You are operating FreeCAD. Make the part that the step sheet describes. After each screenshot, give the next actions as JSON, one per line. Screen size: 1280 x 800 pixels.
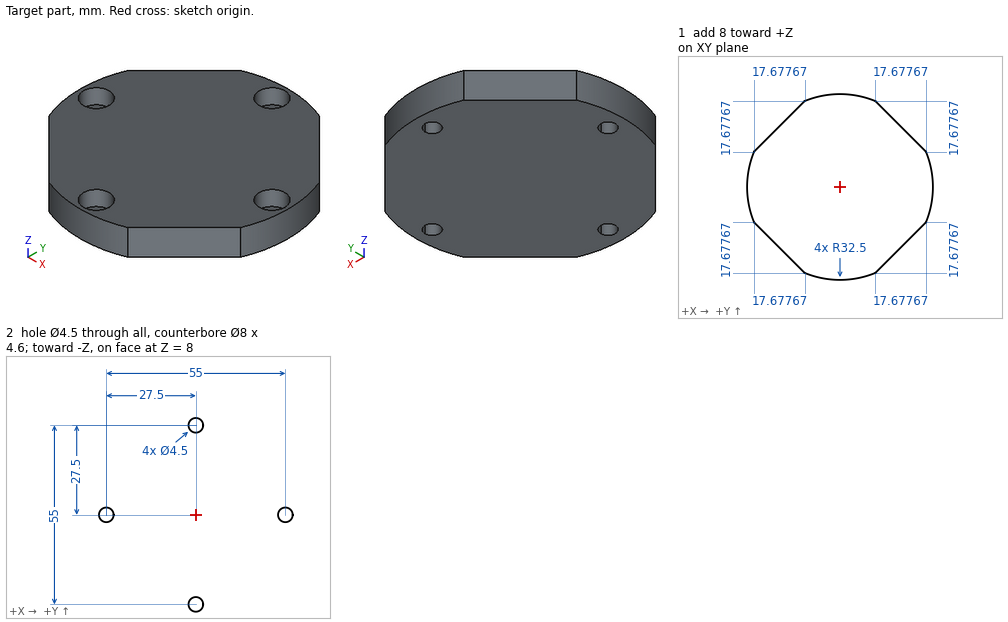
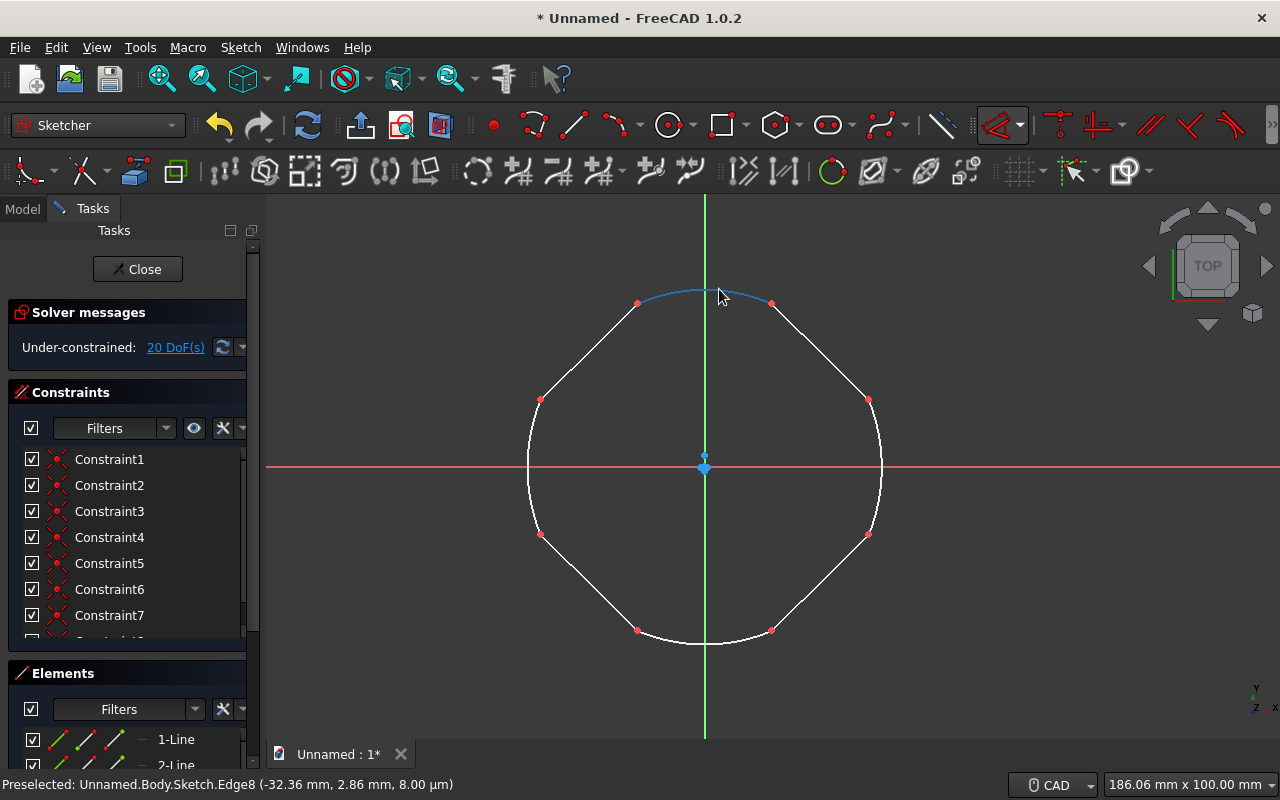
{"action": "left_click", "coordinate": [677, 642]}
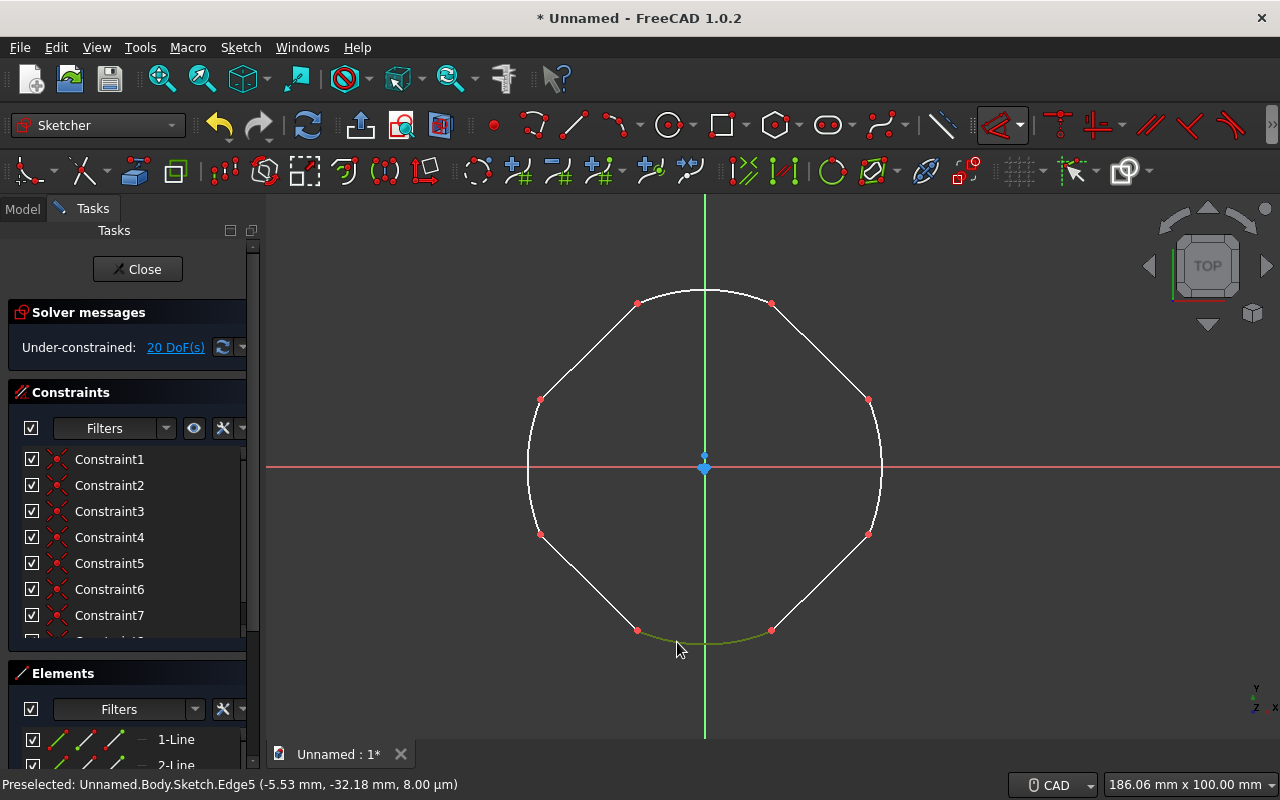
{"action": "left_click", "coordinate": [880, 495]}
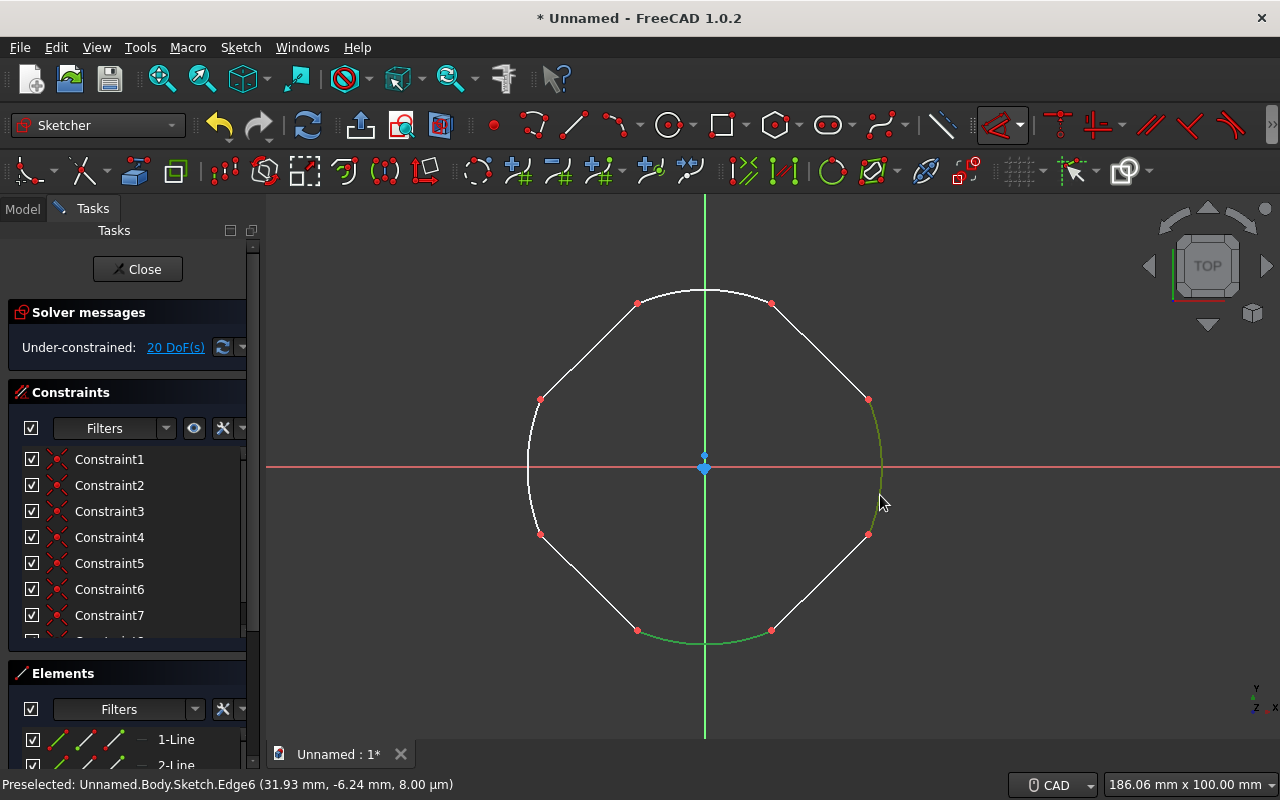
{"action": "left_click", "coordinate": [1058, 126]}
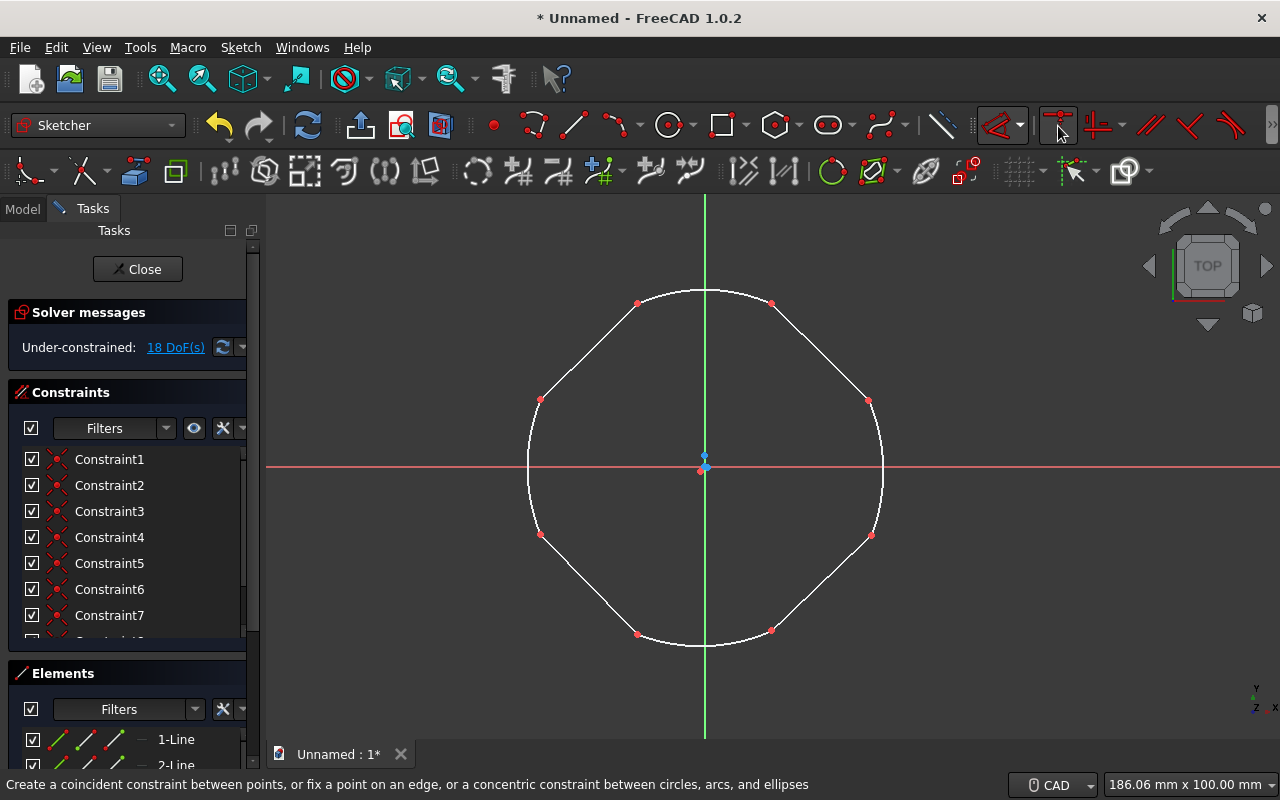
{"action": "left_click", "coordinate": [678, 645]}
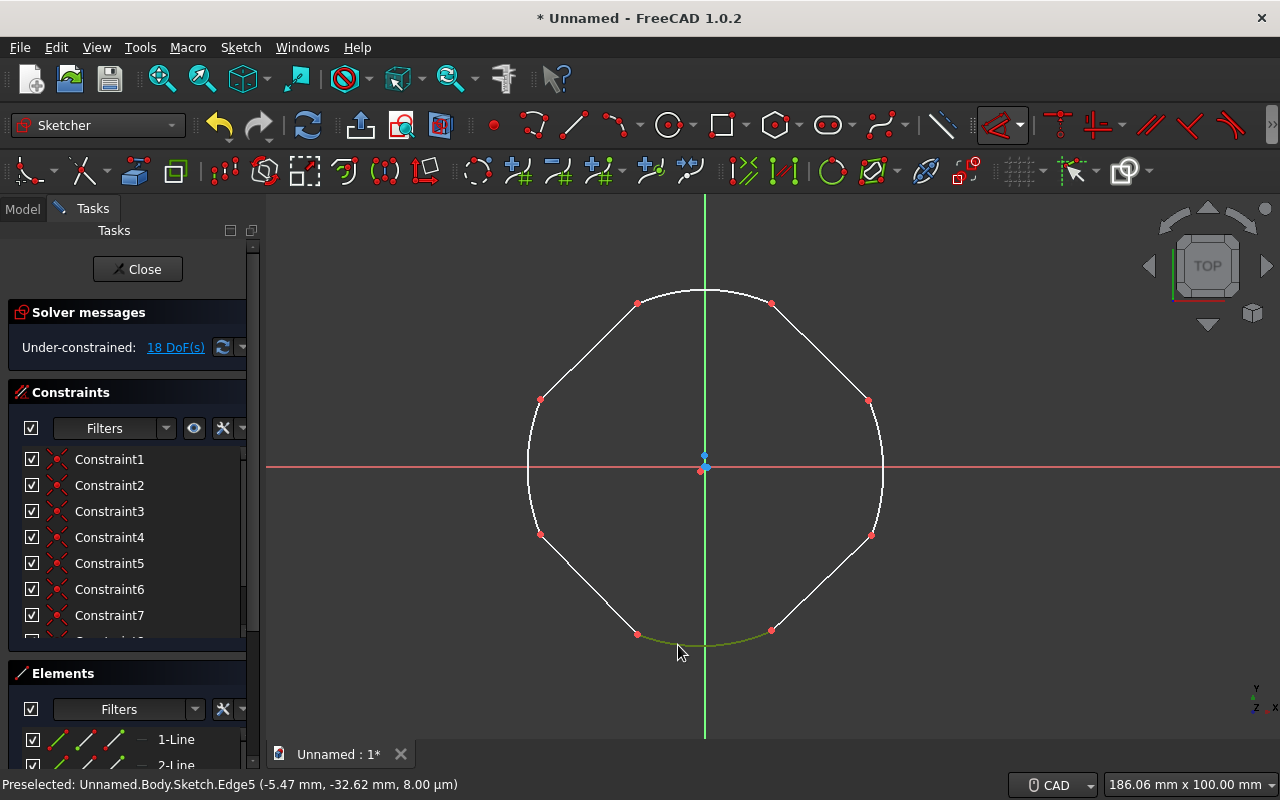
{"action": "left_click", "coordinate": [732, 292]}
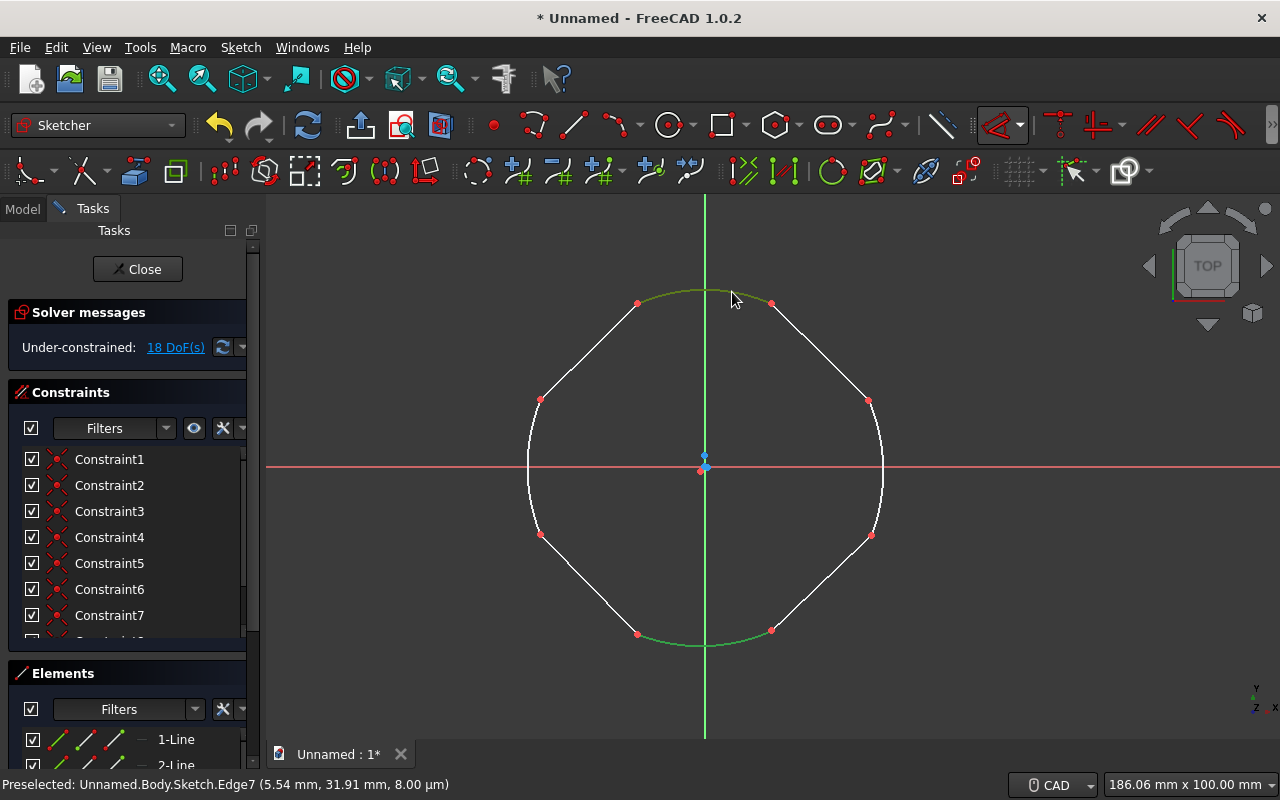
{"action": "key", "text": "c"}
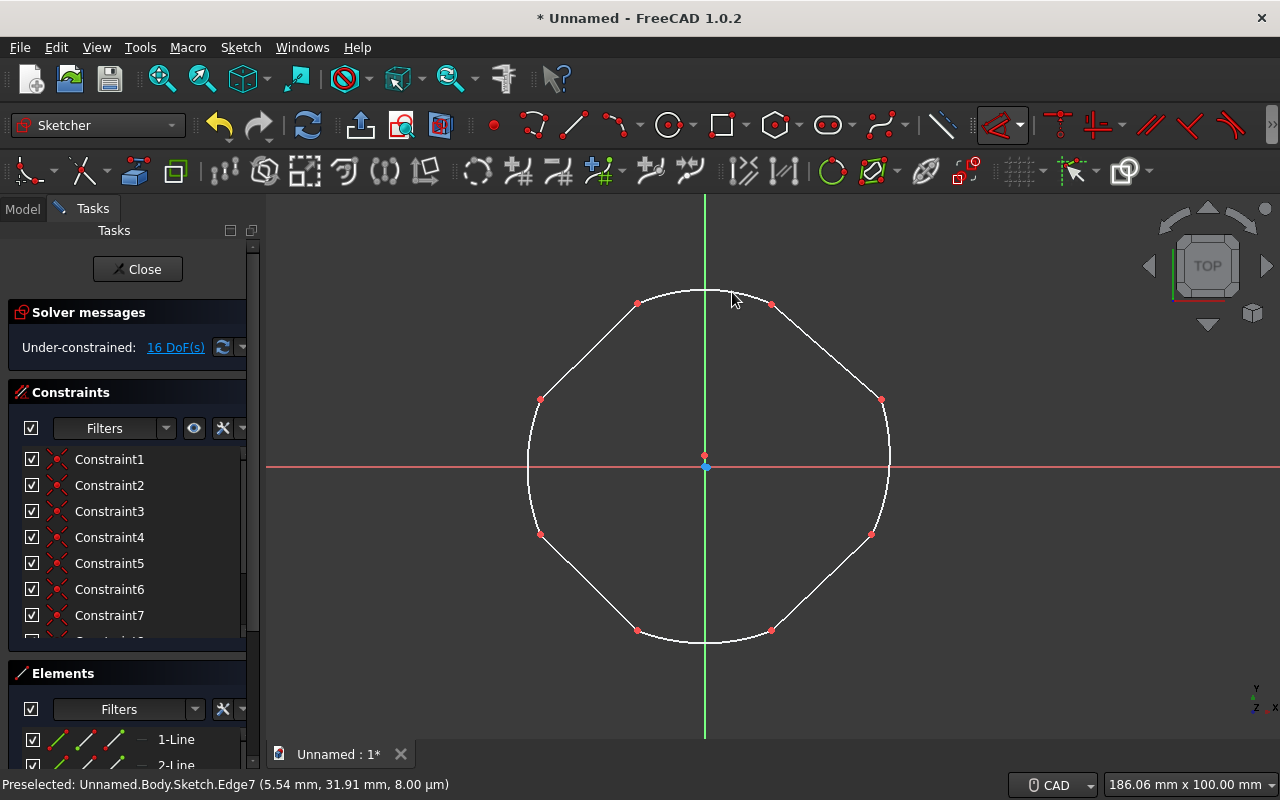
{"action": "left_click", "coordinate": [677, 641]}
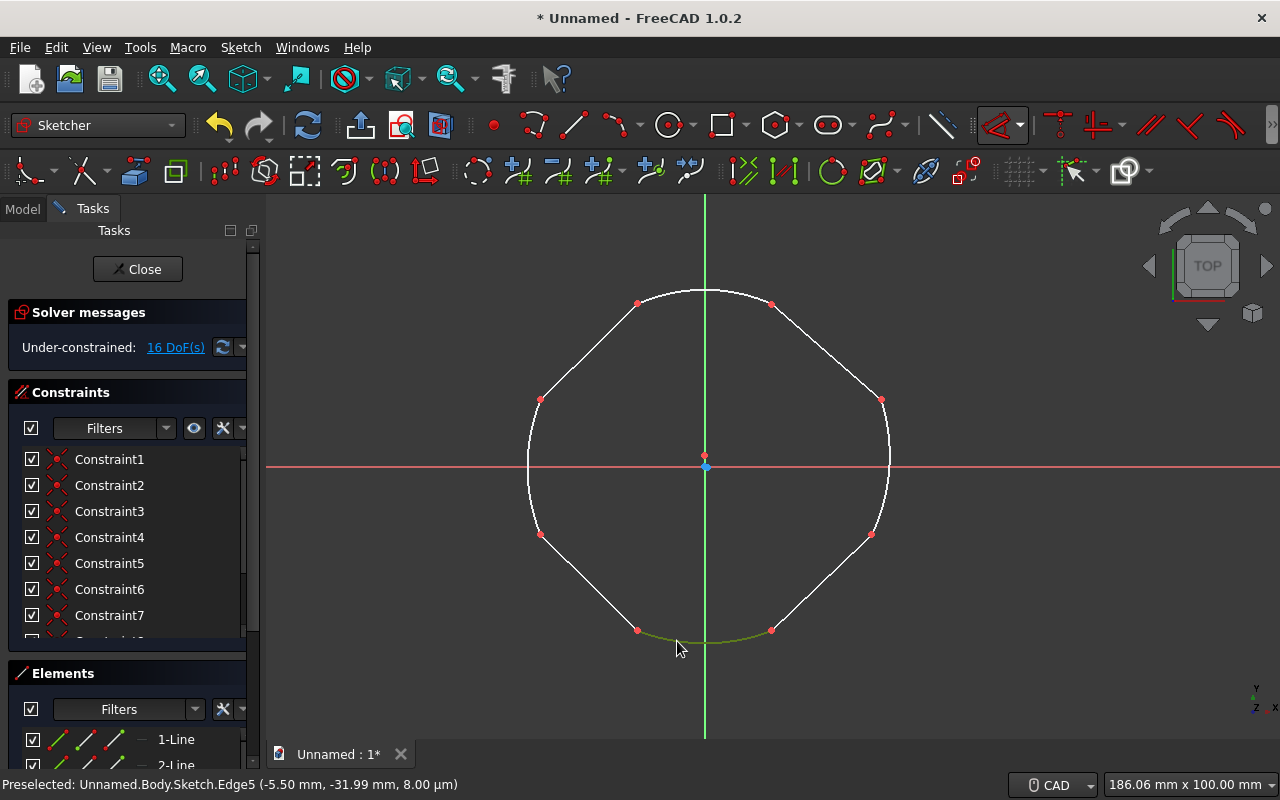
{"action": "left_click", "coordinate": [530, 440]}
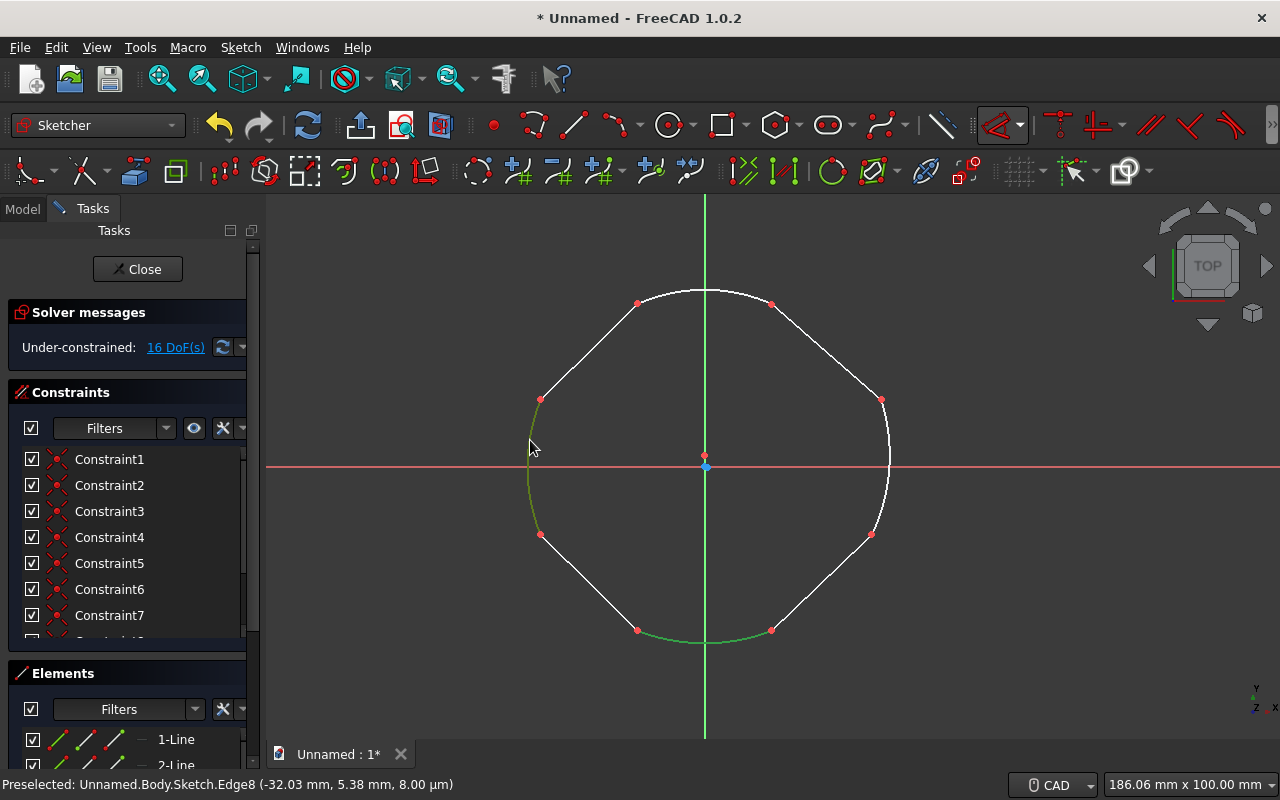
{"action": "left_click", "coordinate": [1058, 126]}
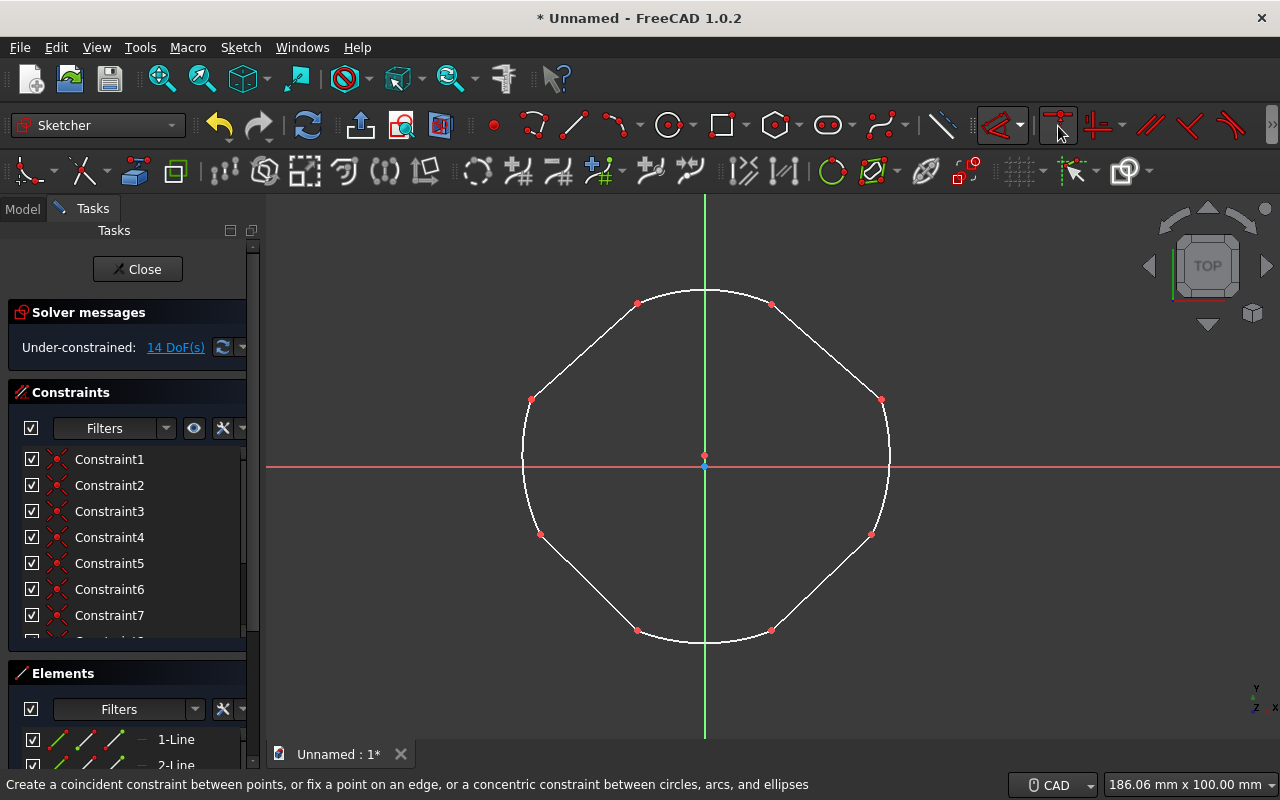
{"action": "left_click_drag", "start_coordinate": [695, 446], "coordinate": [715, 476]}